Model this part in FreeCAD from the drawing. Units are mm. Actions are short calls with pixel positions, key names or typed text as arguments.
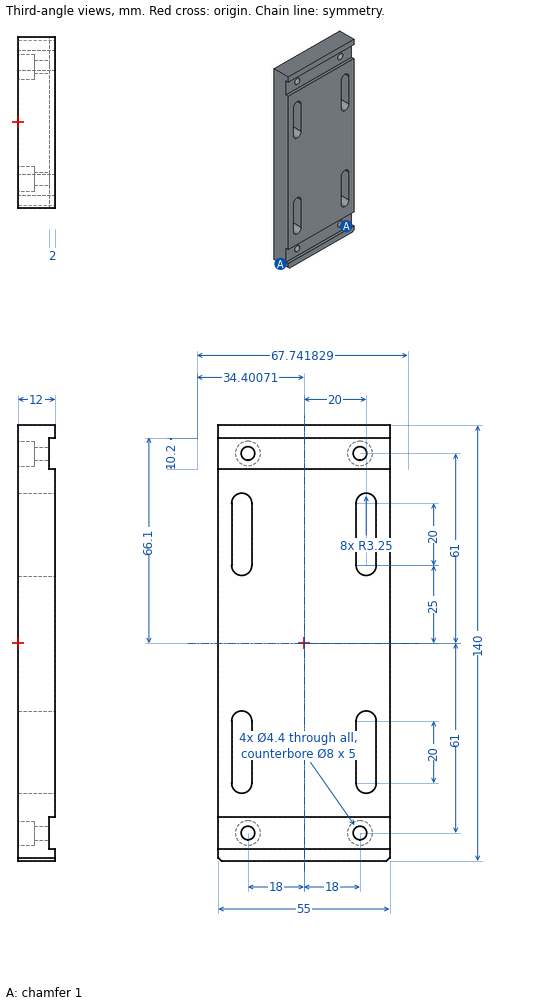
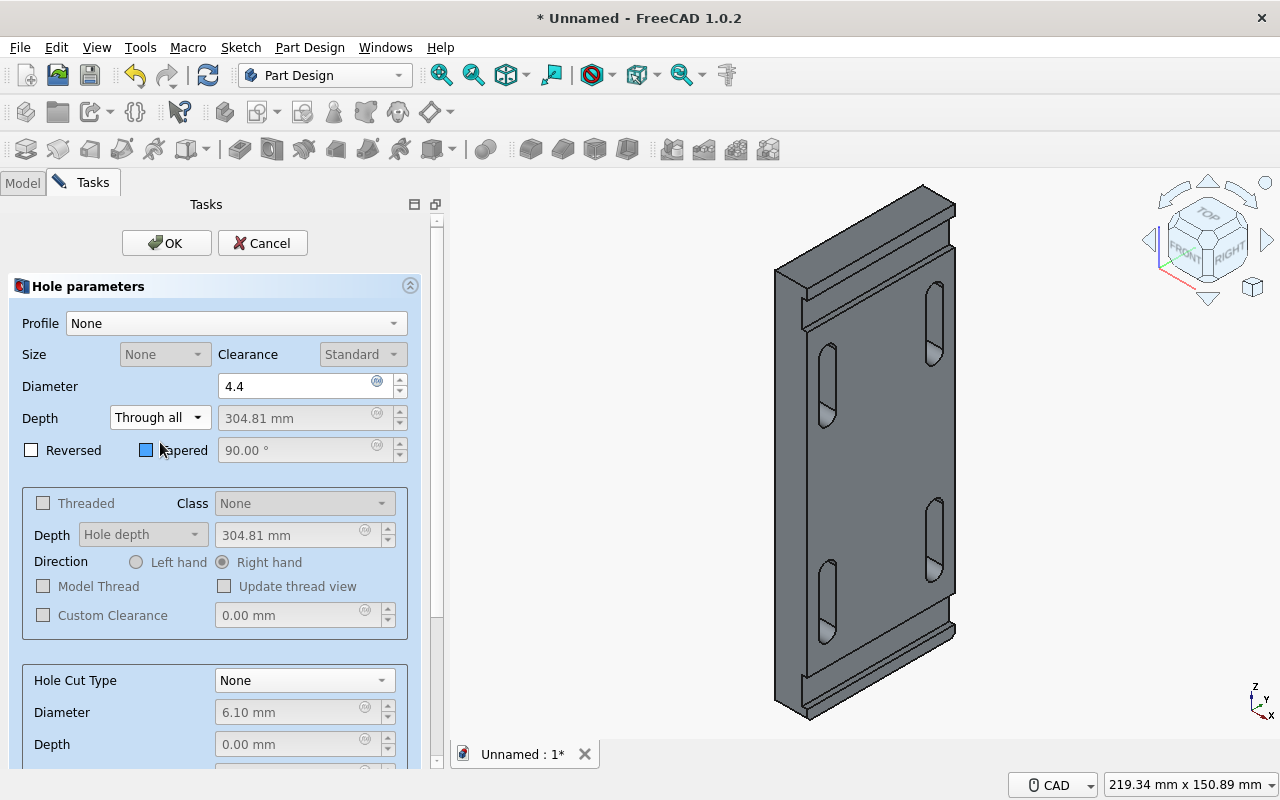
click(30, 450)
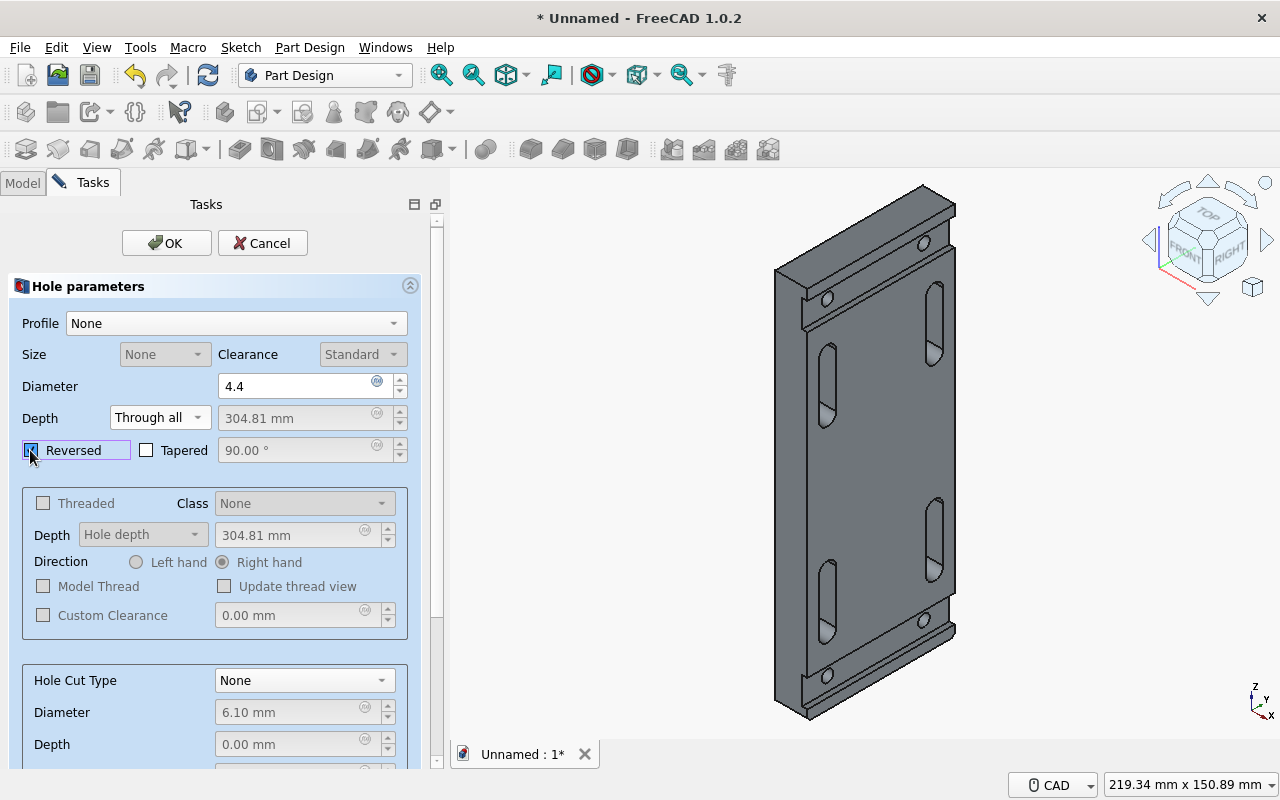
click(306, 680)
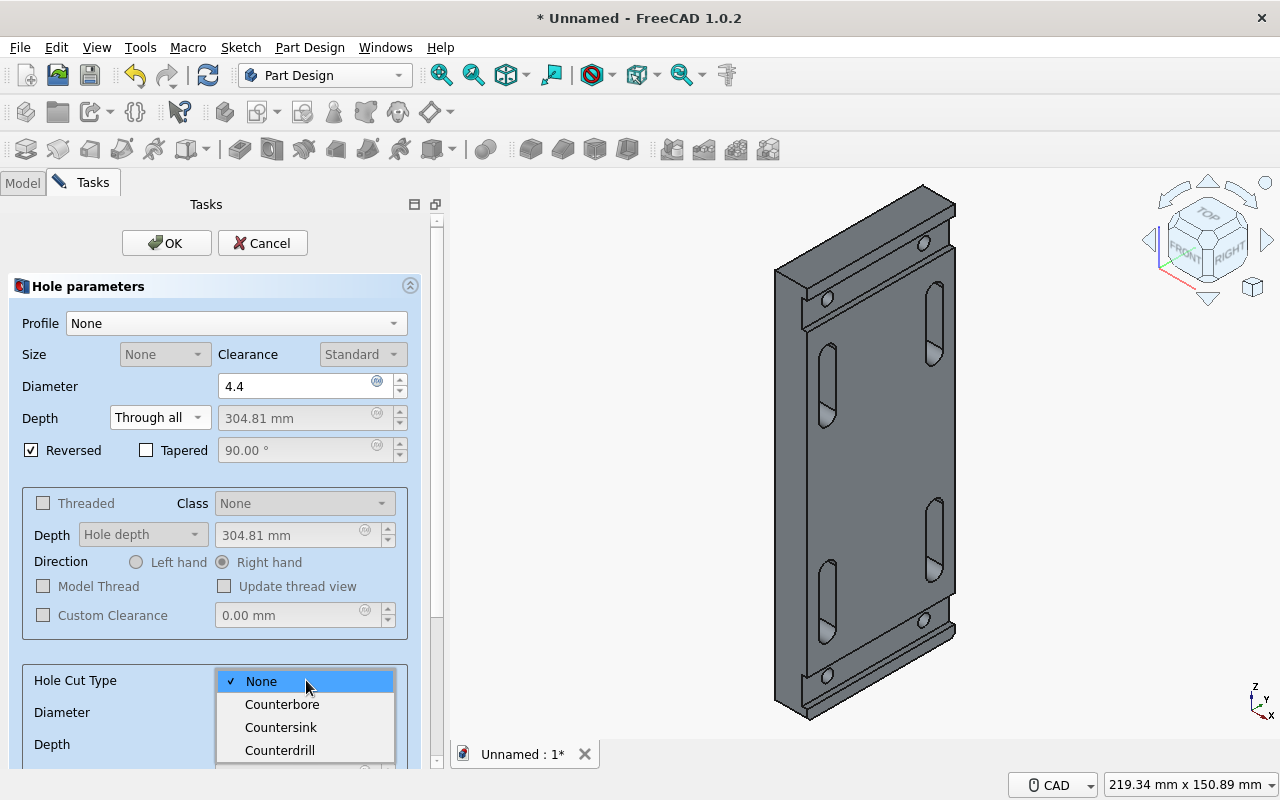
click(304, 704)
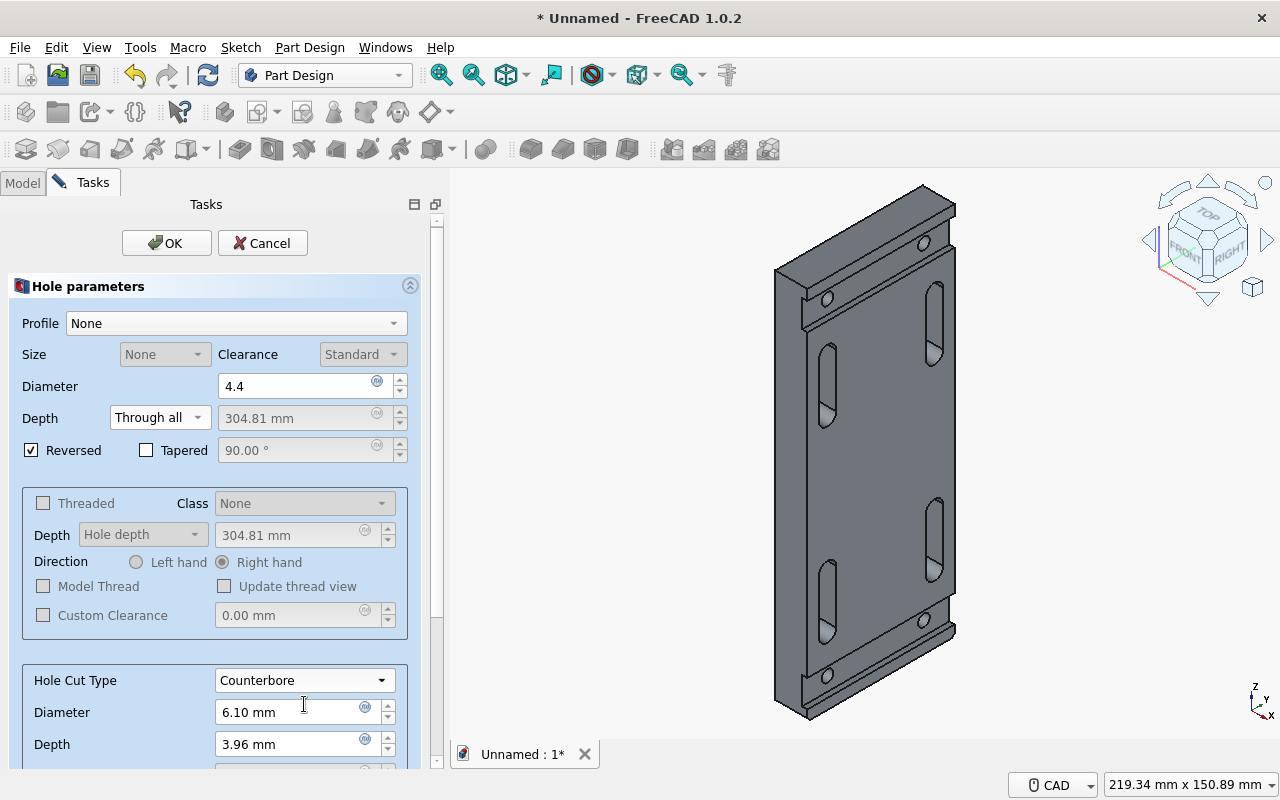
triple_click(298, 712)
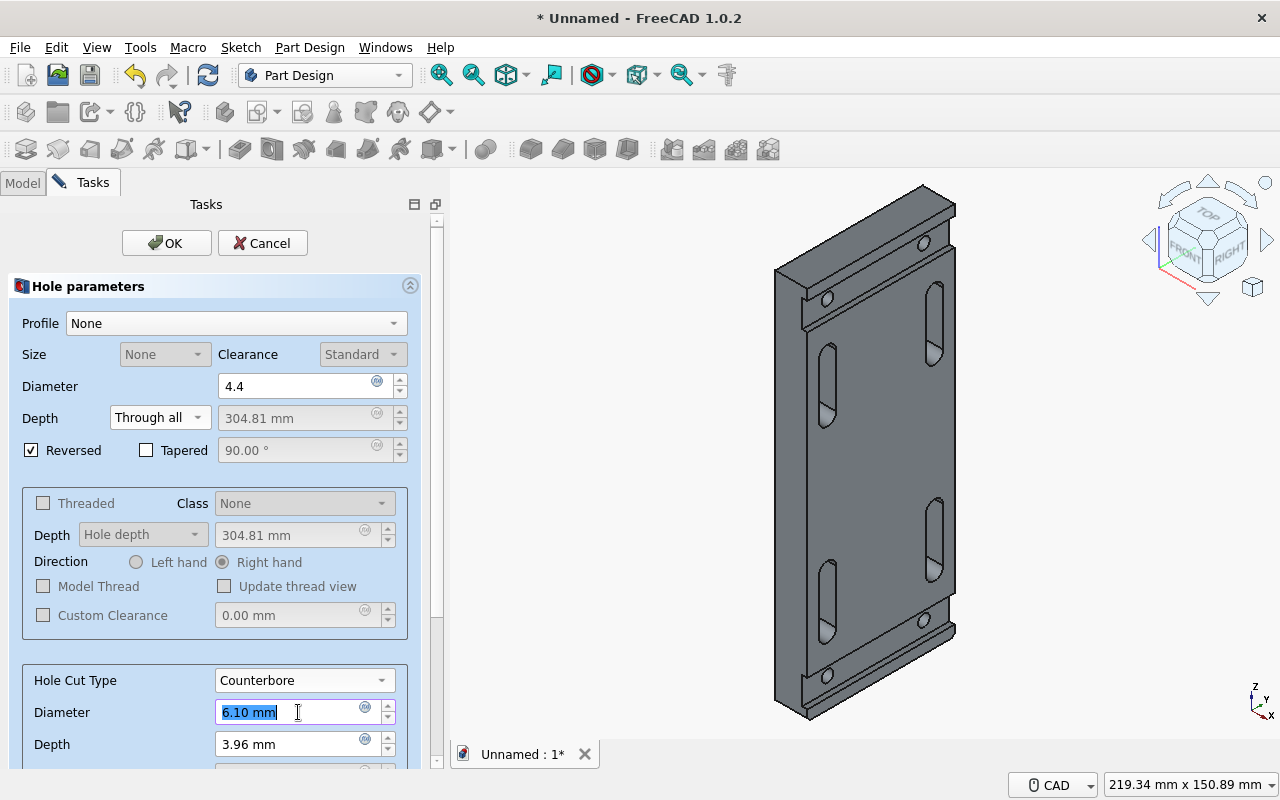
text(8)
key(Tab)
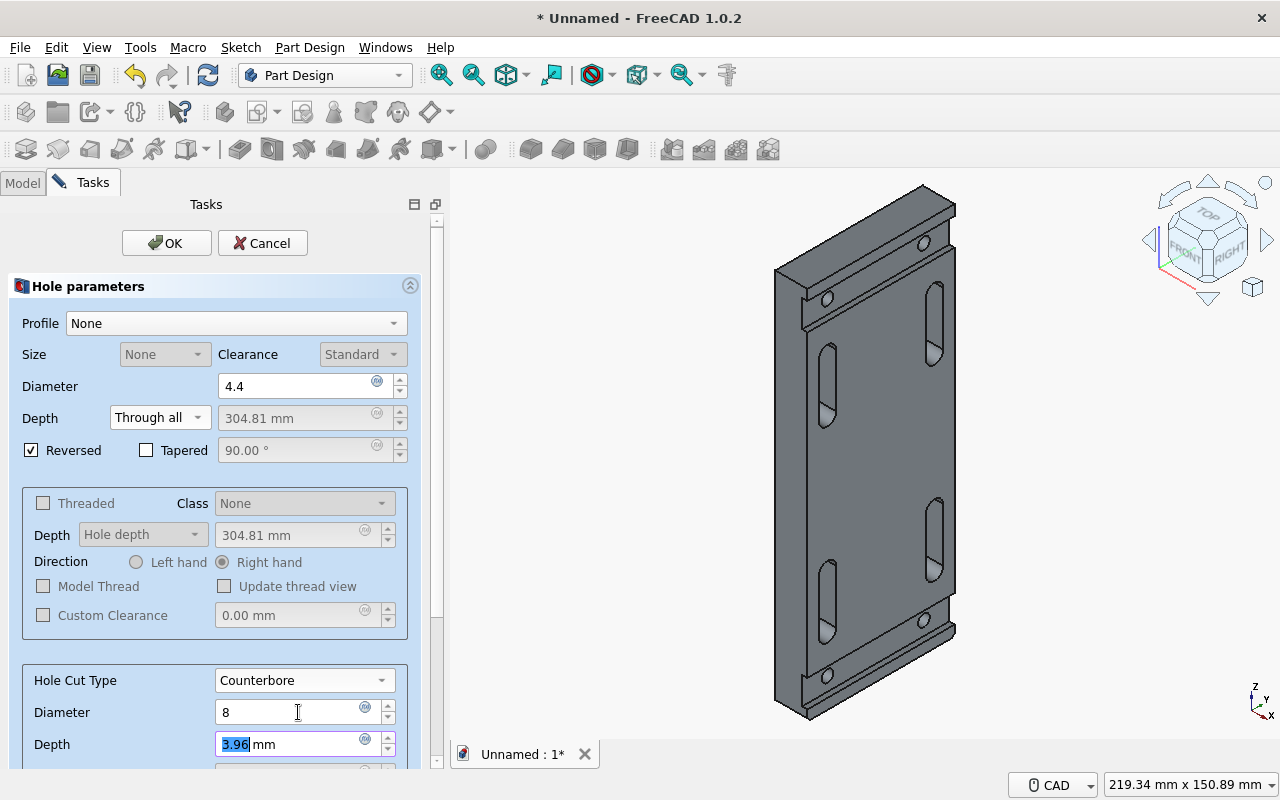
text(5)
key(Tab)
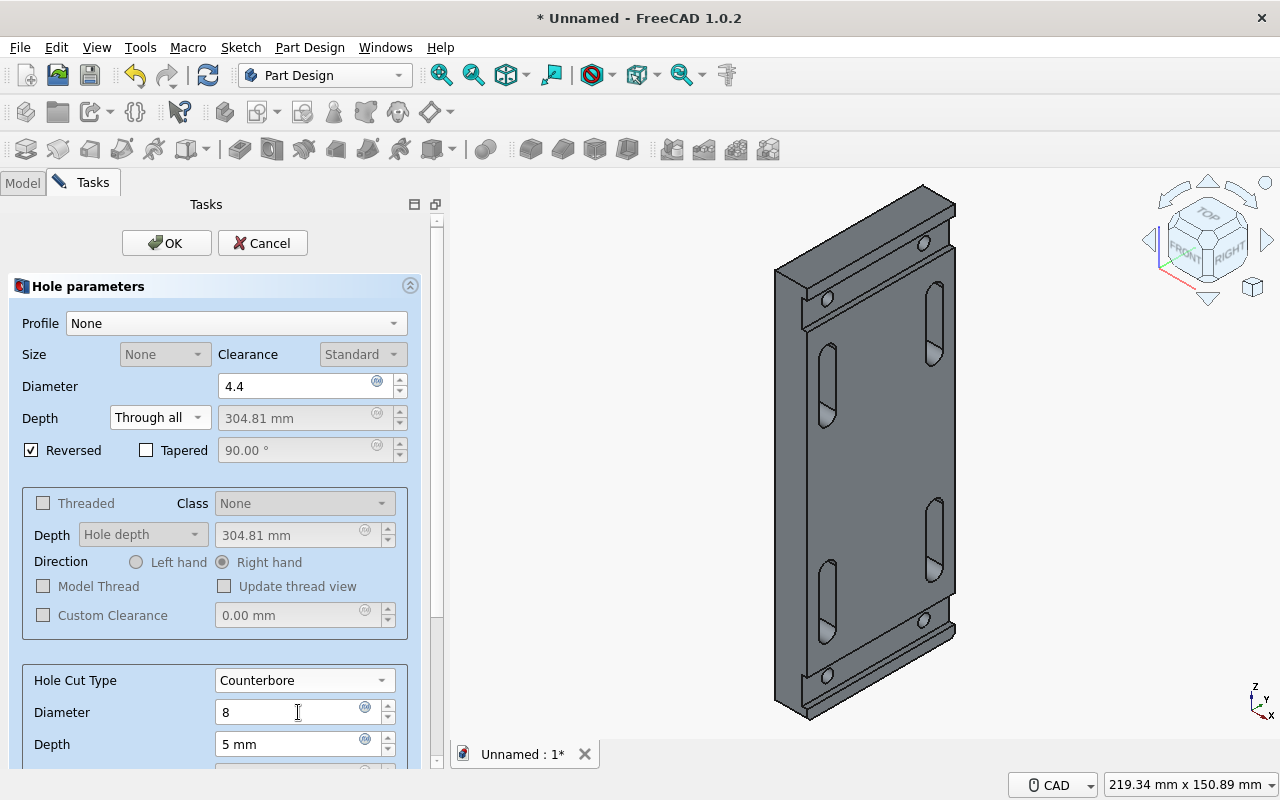
click(167, 243)